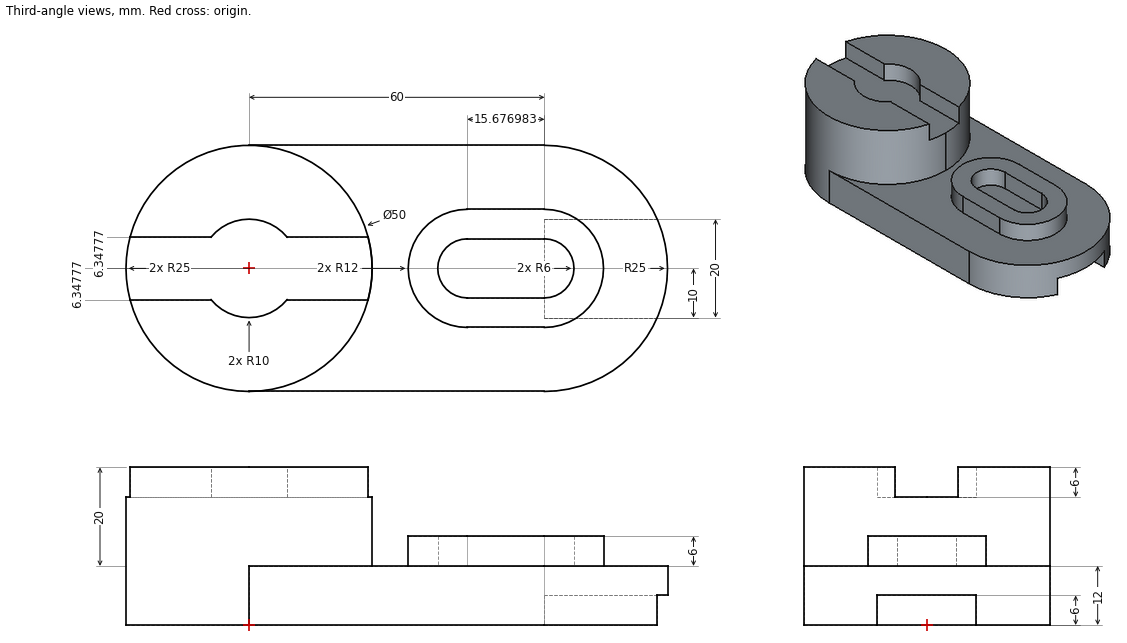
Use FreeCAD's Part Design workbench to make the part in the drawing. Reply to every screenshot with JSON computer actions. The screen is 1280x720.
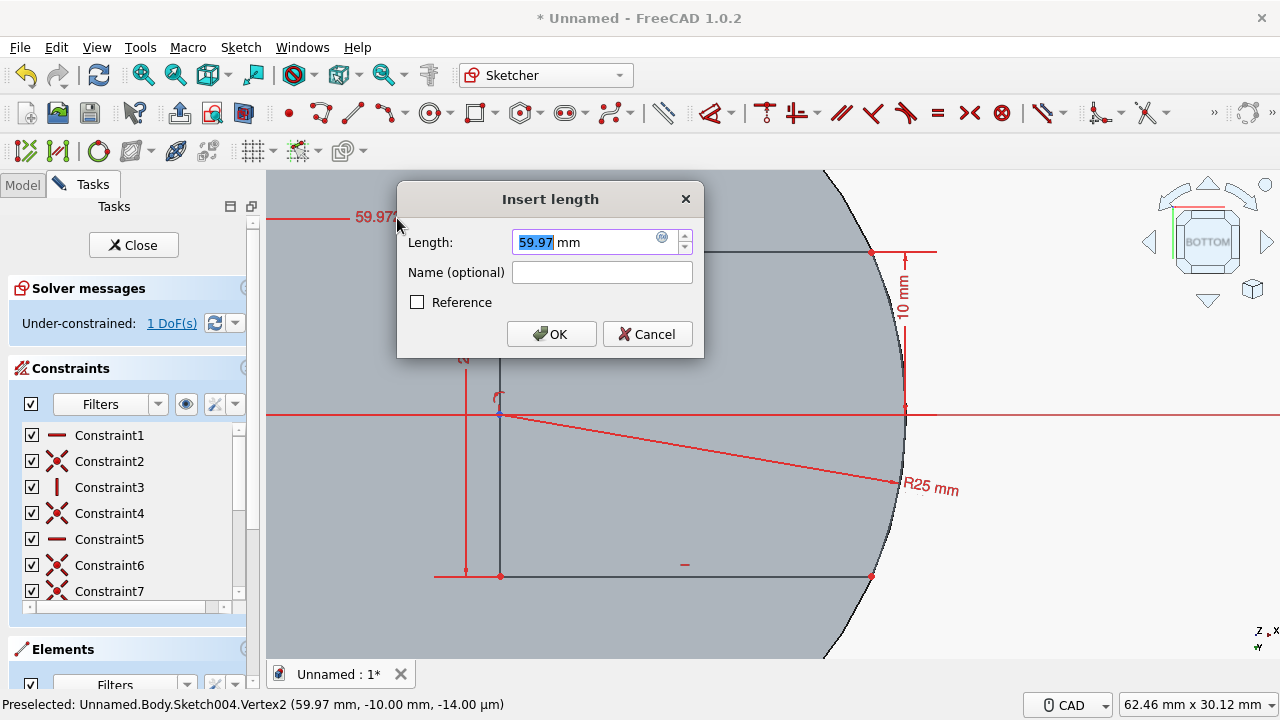
{"action": "type", "text": "60"}
{"action": "key", "text": "Return"}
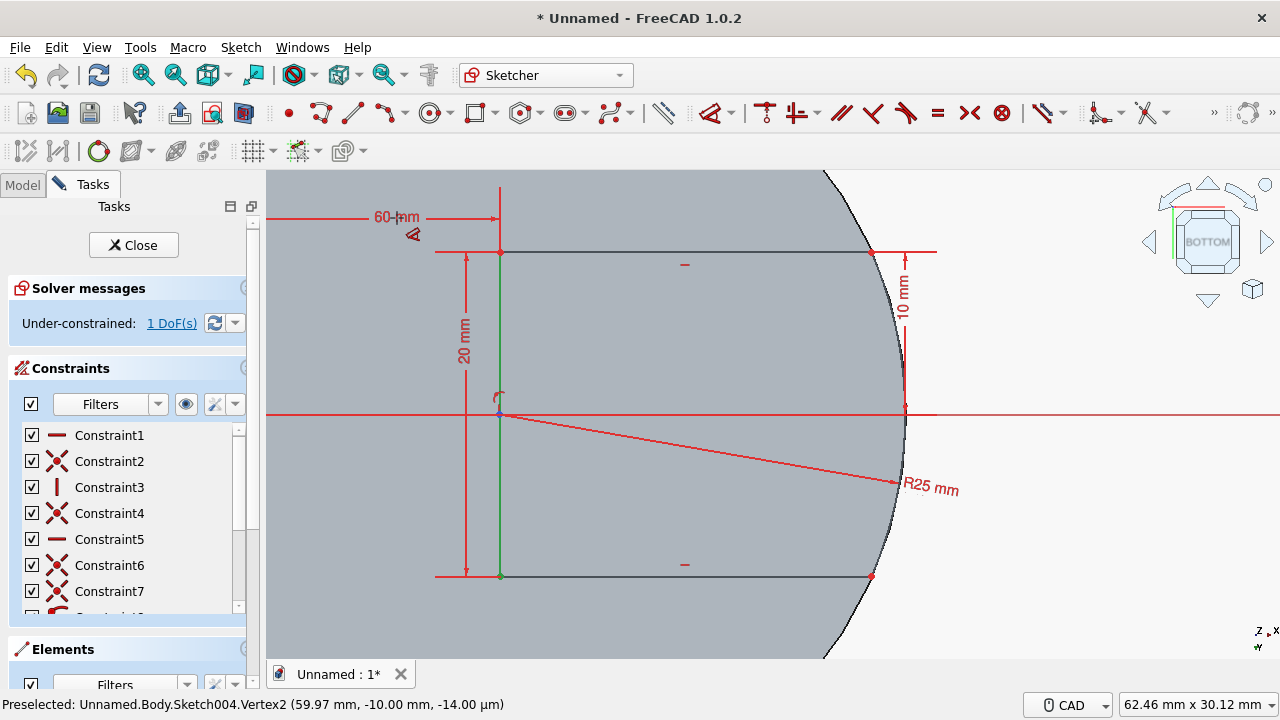
{"action": "left_click", "coordinate": [499, 414]}
{"action": "left_click", "coordinate": [397, 448]}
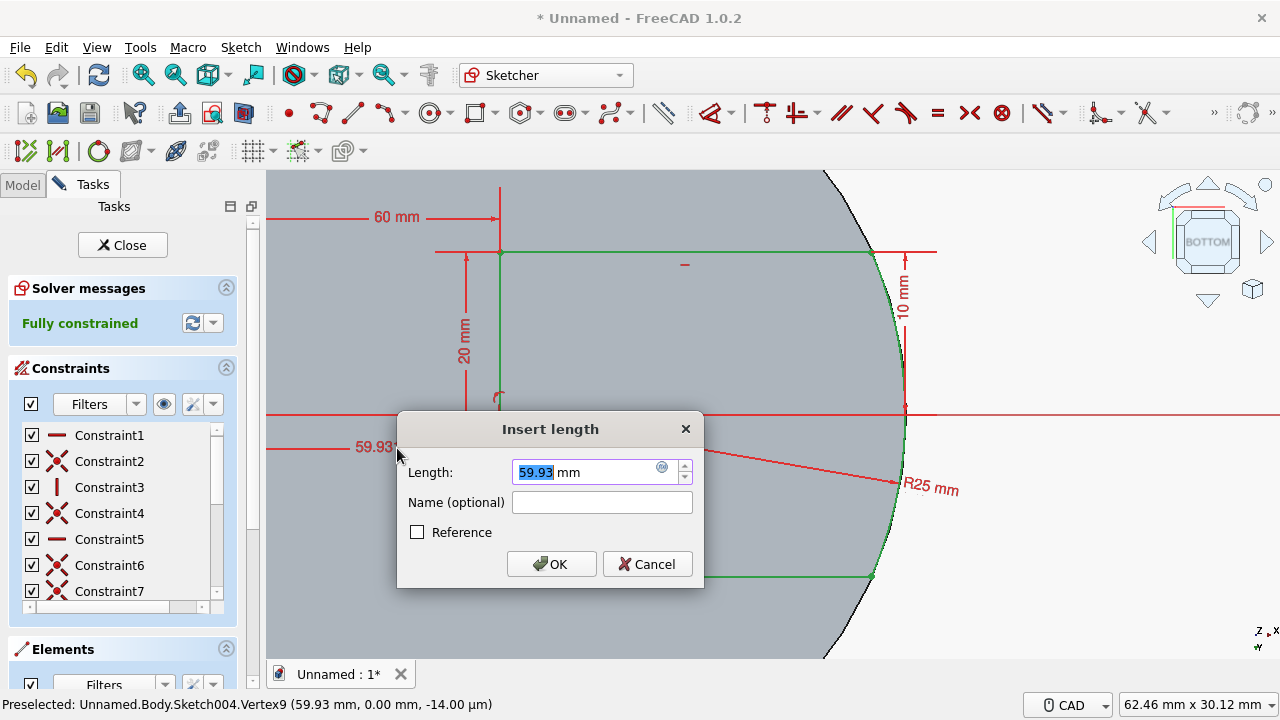
{"action": "type", "text": "60"}
{"action": "key", "text": "Return"}
{"action": "key", "text": "Escape"}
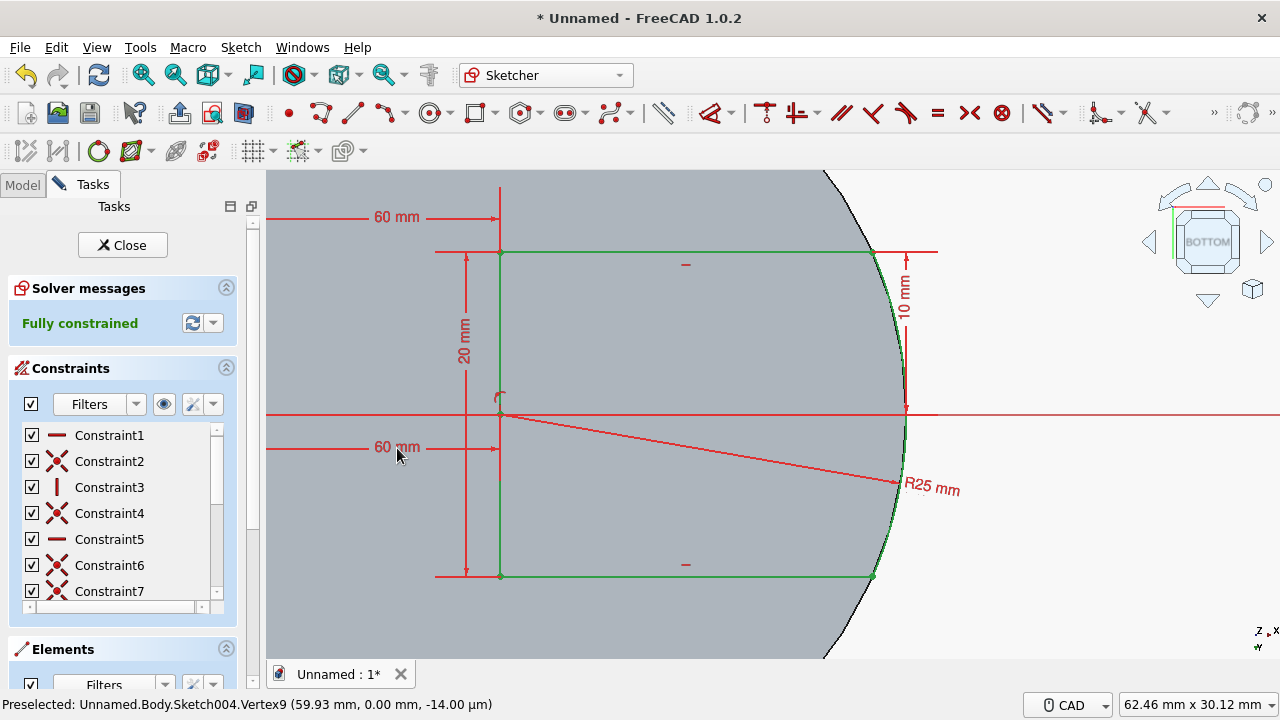
{"action": "left_click", "coordinate": [123, 245]}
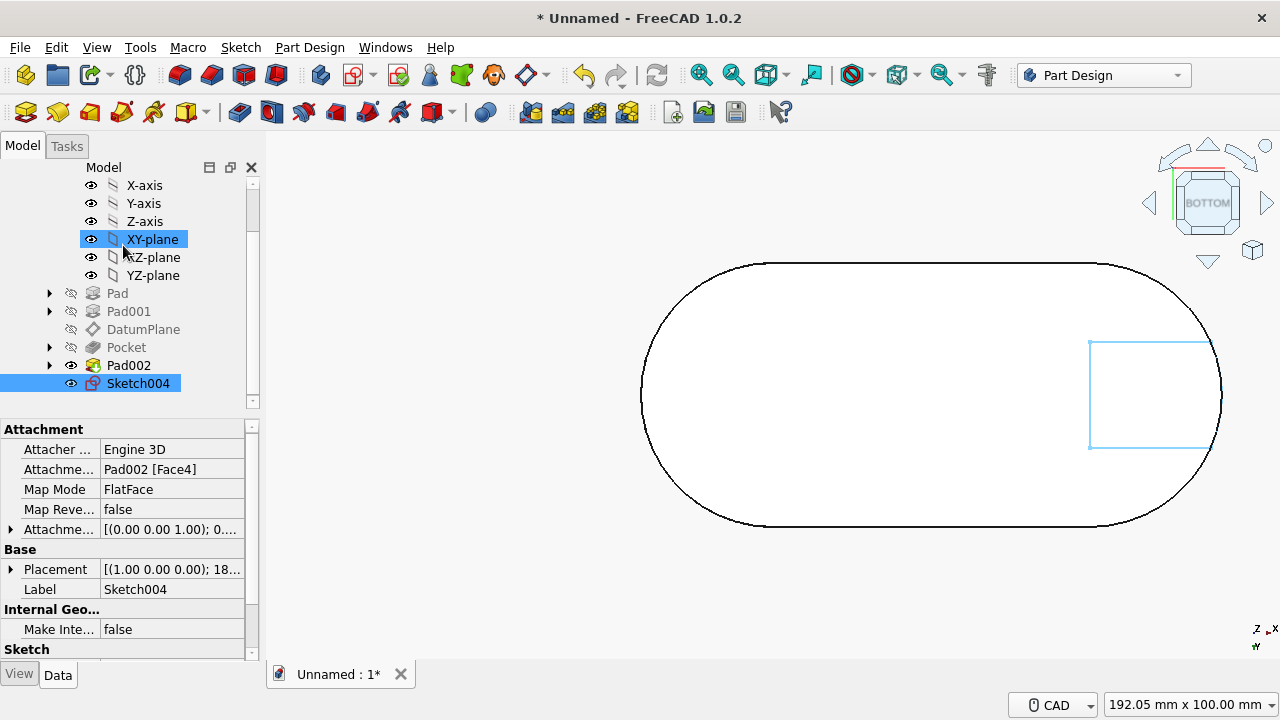
{"action": "left_click", "coordinate": [240, 112]}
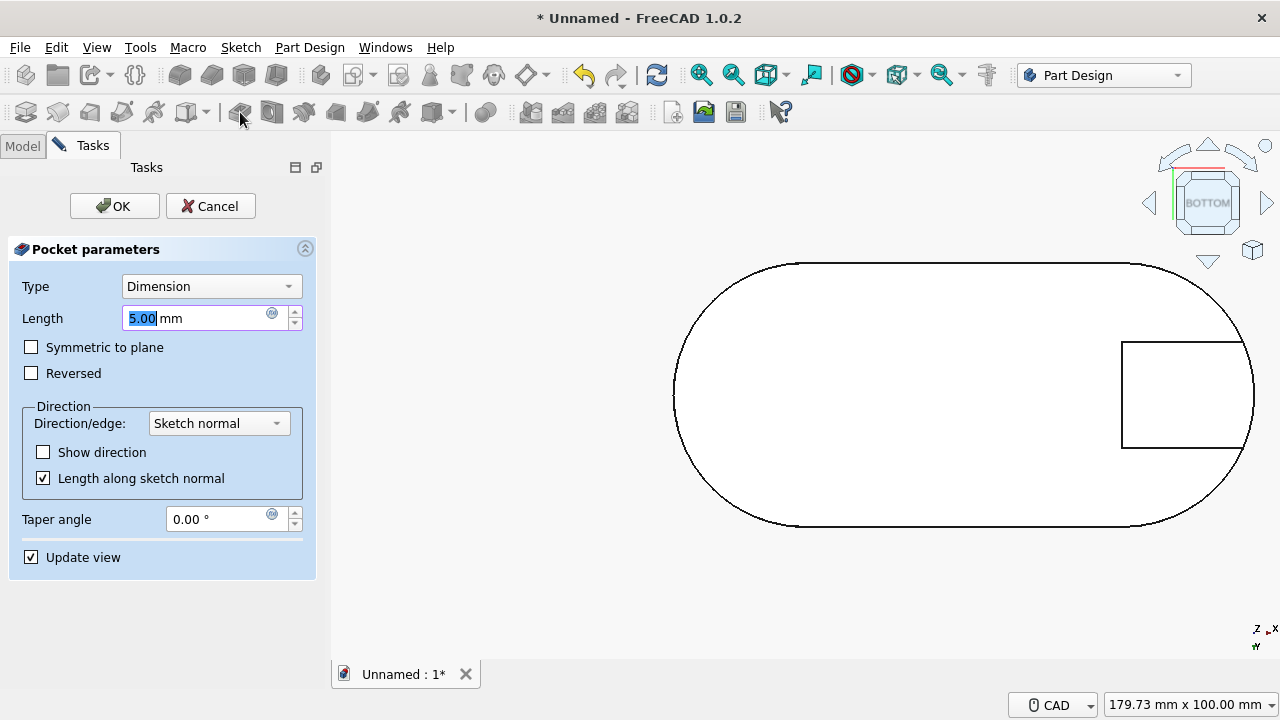
{"action": "left_click", "coordinate": [212, 286]}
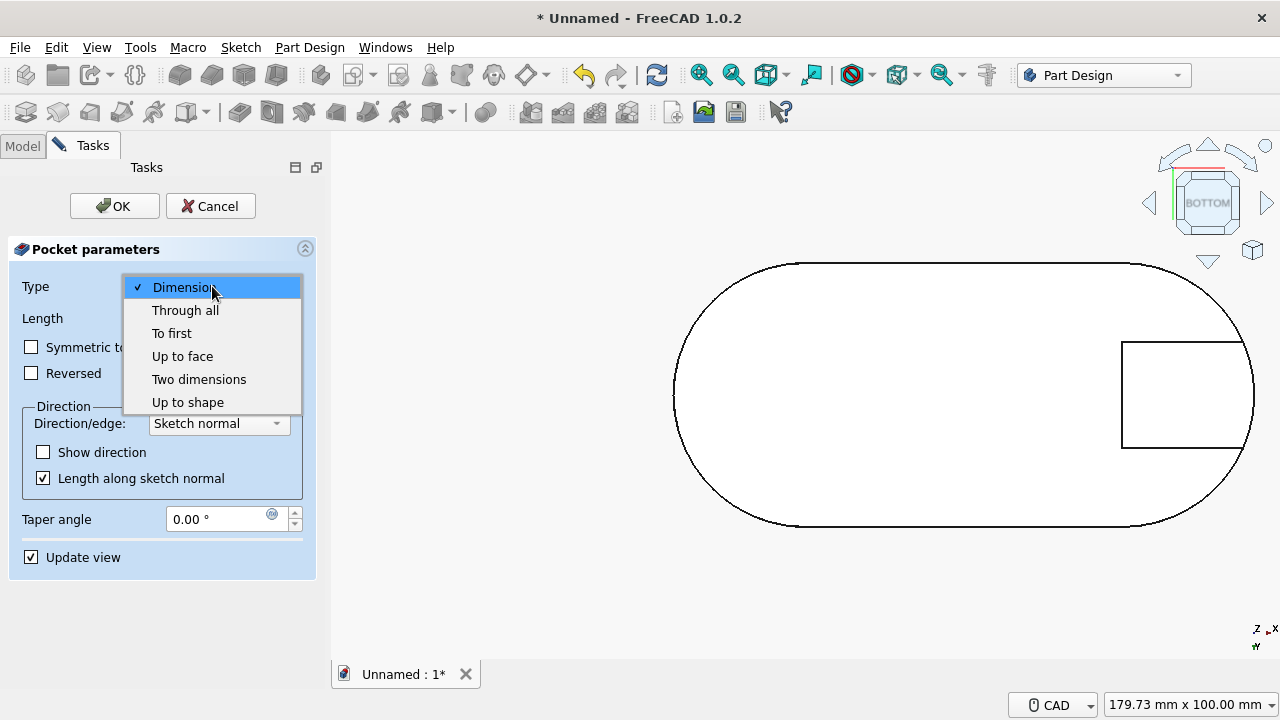
{"action": "left_click", "coordinate": [212, 380]}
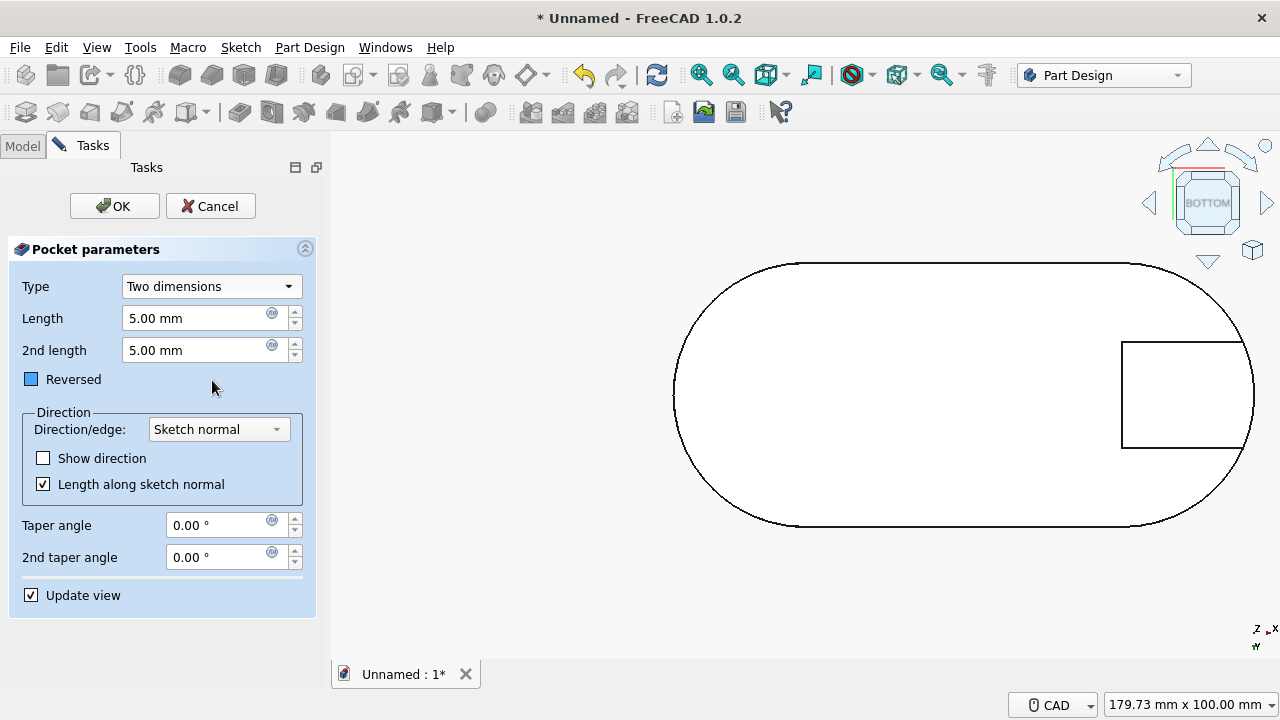
{"action": "triple_click", "coordinate": [204, 318]}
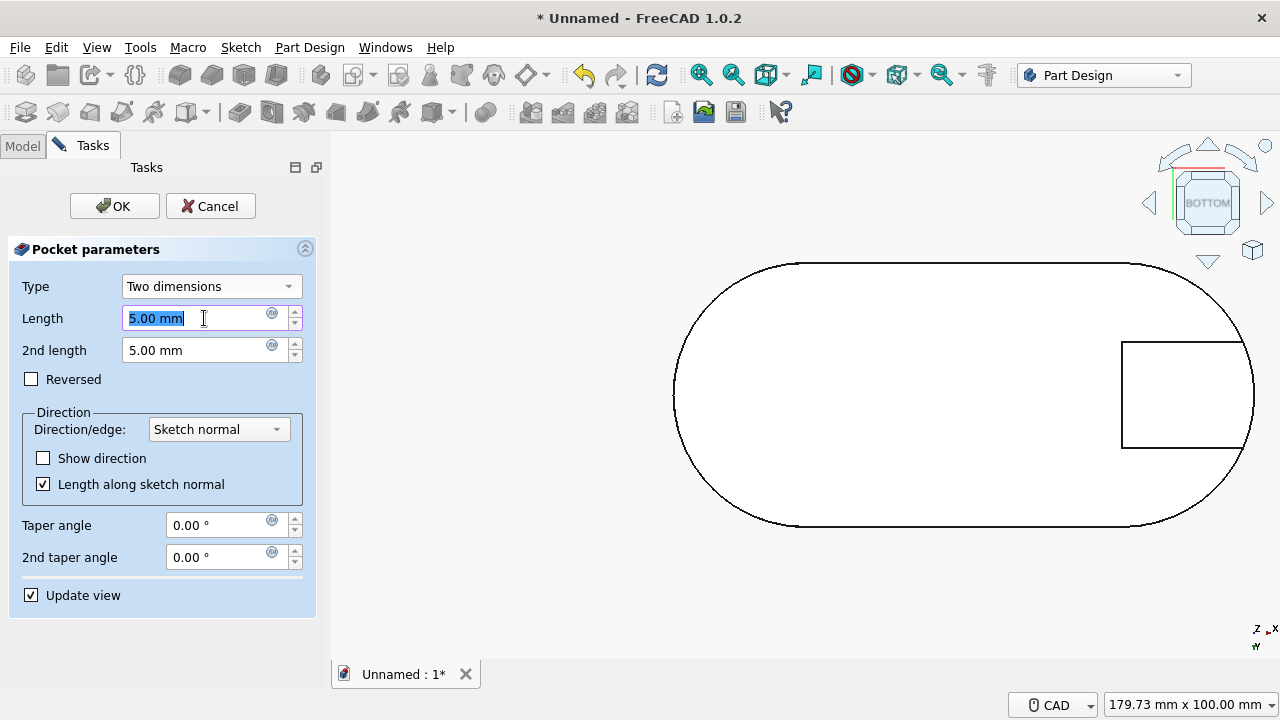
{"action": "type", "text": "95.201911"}
{"action": "key", "text": "Tab"}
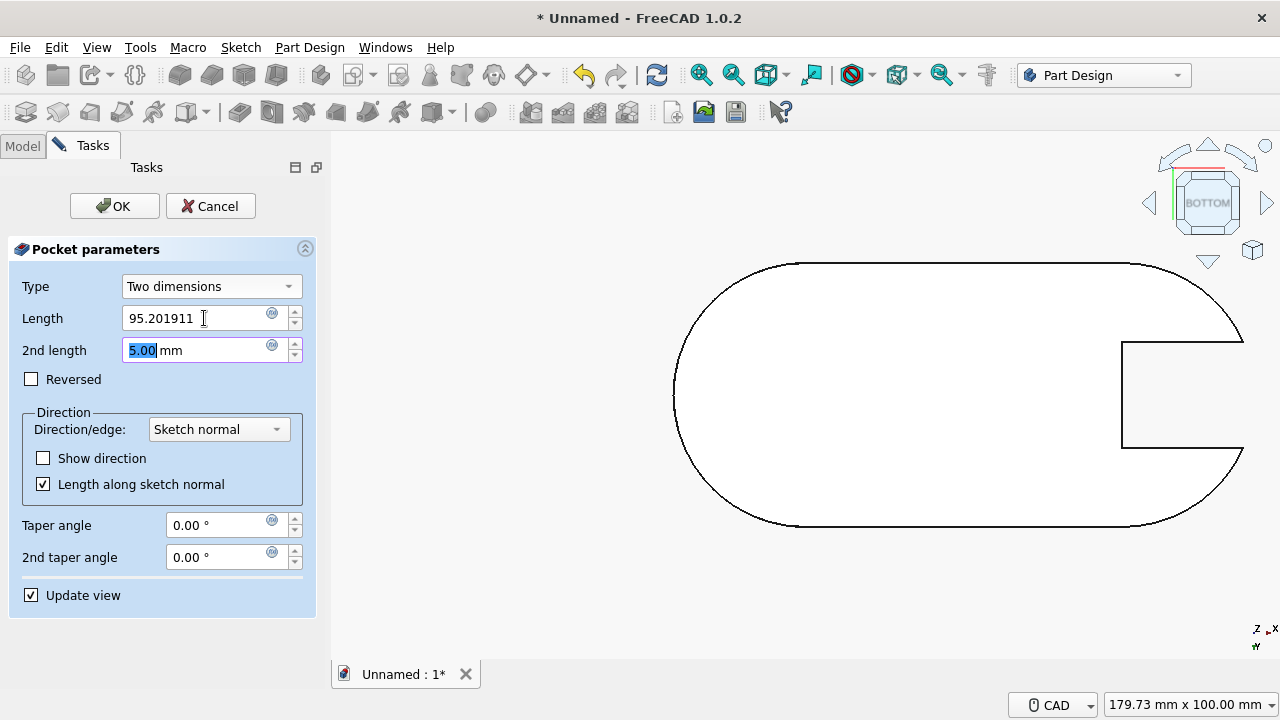
{"action": "type", "text": "6"}
{"action": "key", "text": "Tab"}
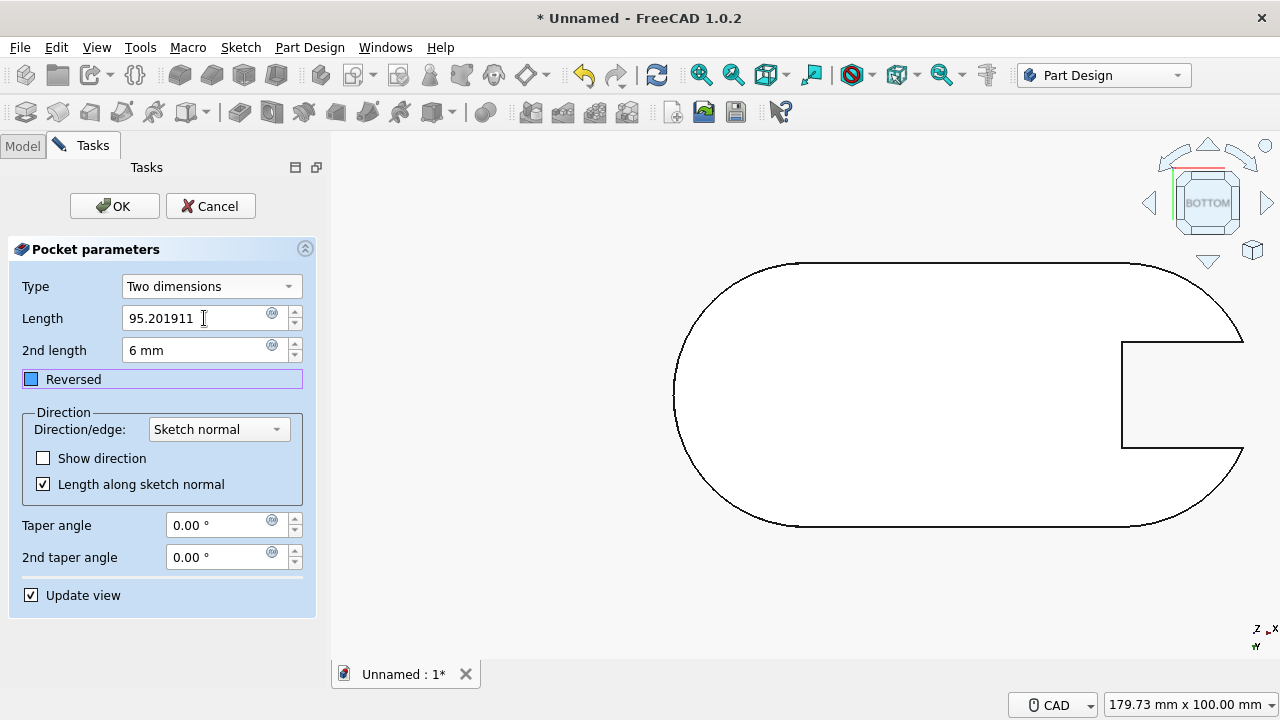
{"action": "left_click", "coordinate": [30, 379]}